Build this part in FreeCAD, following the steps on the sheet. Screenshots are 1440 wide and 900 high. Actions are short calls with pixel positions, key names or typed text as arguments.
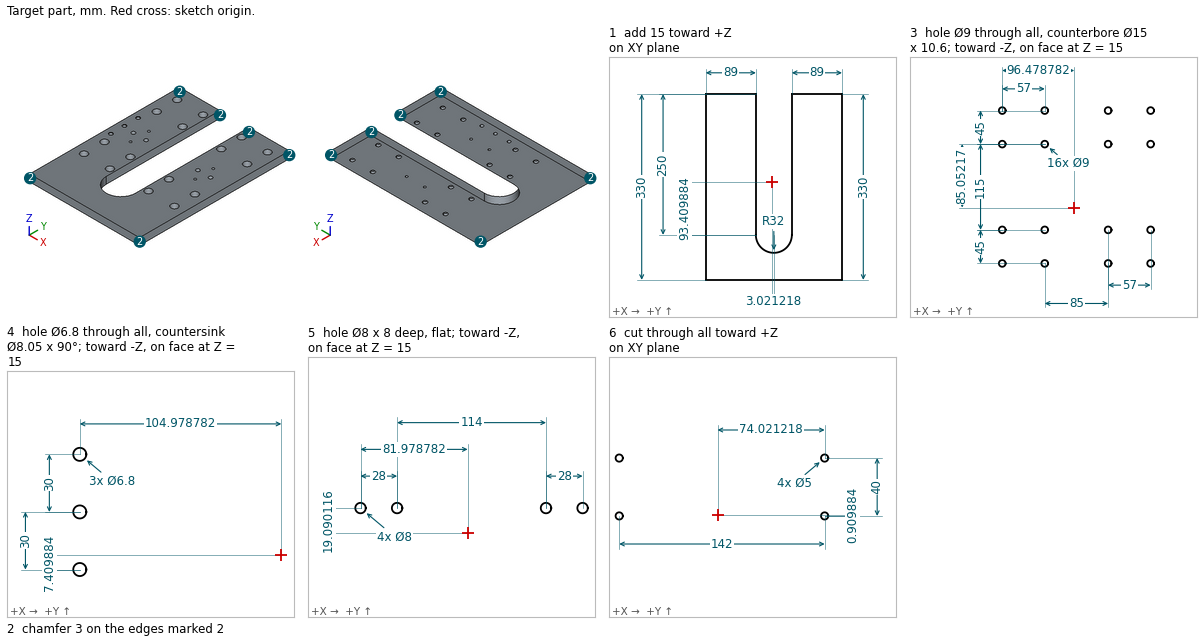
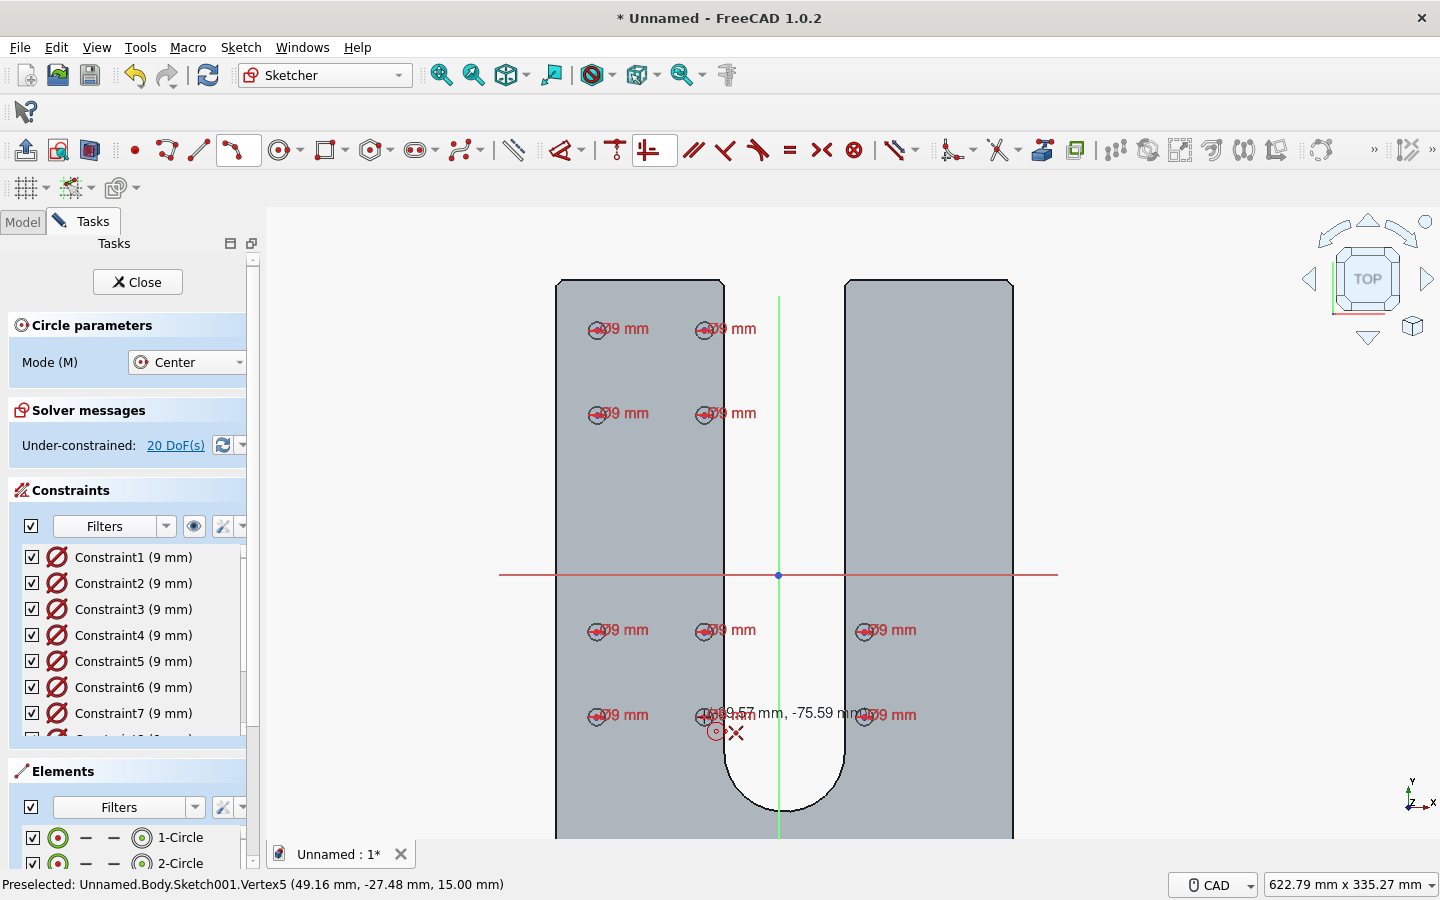
scroll(972, 632, up, 5)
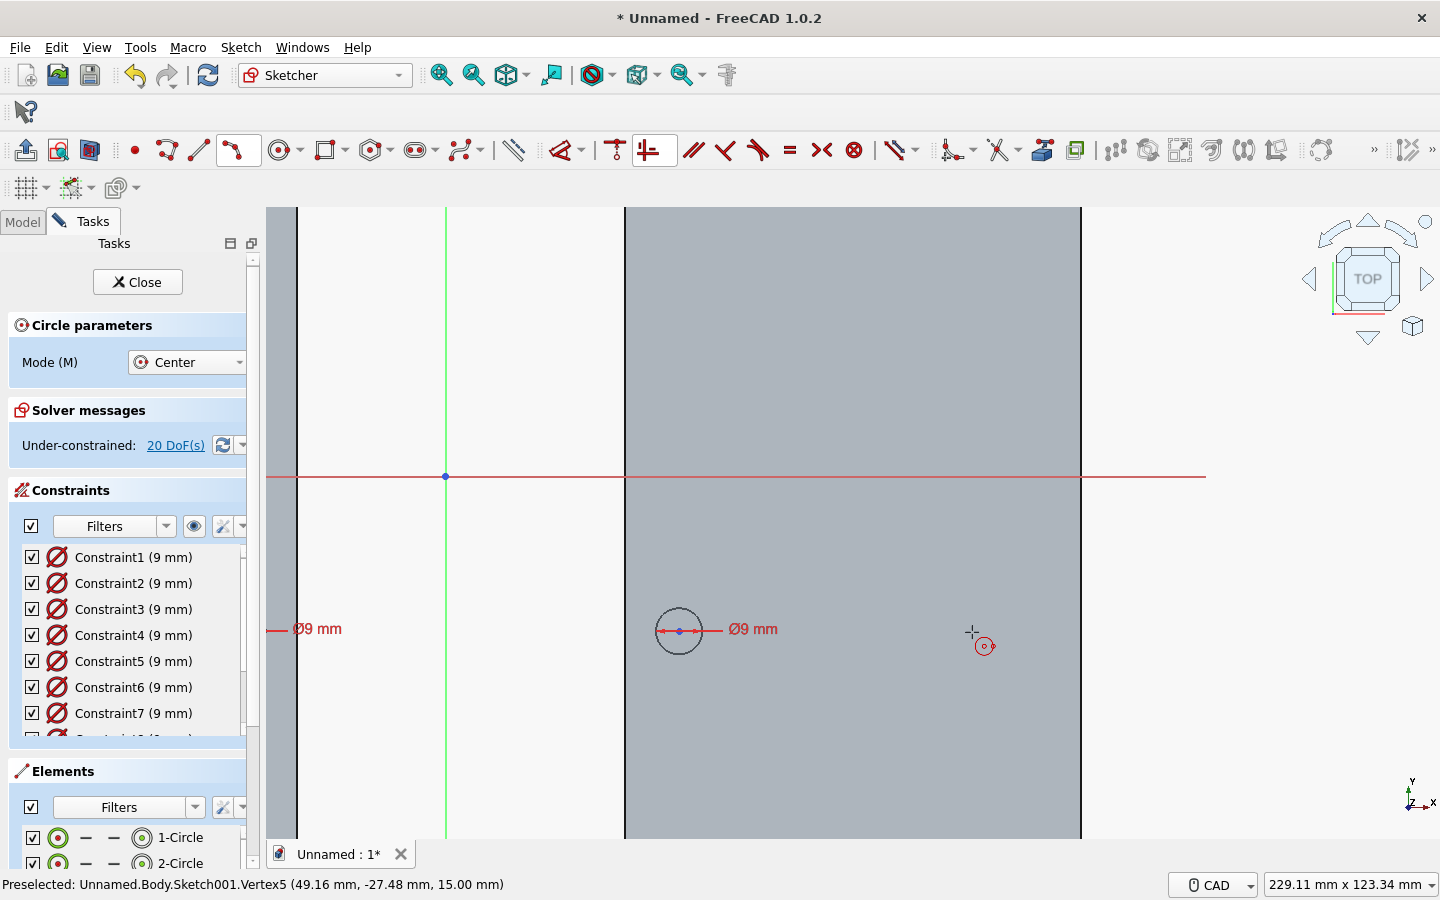
click(971, 630)
move(988, 614)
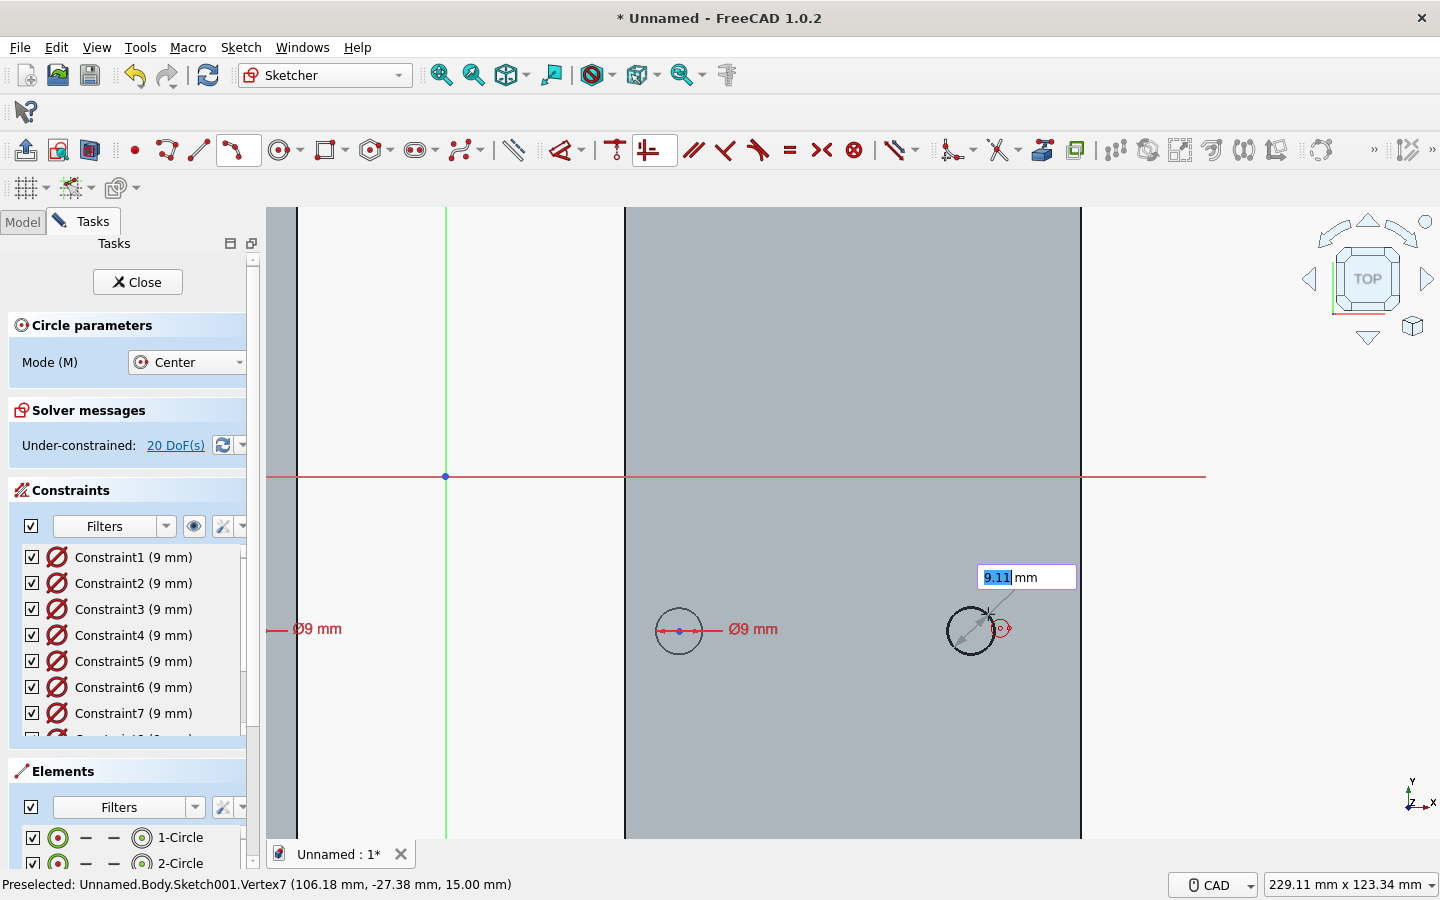
text(9)
key(Return)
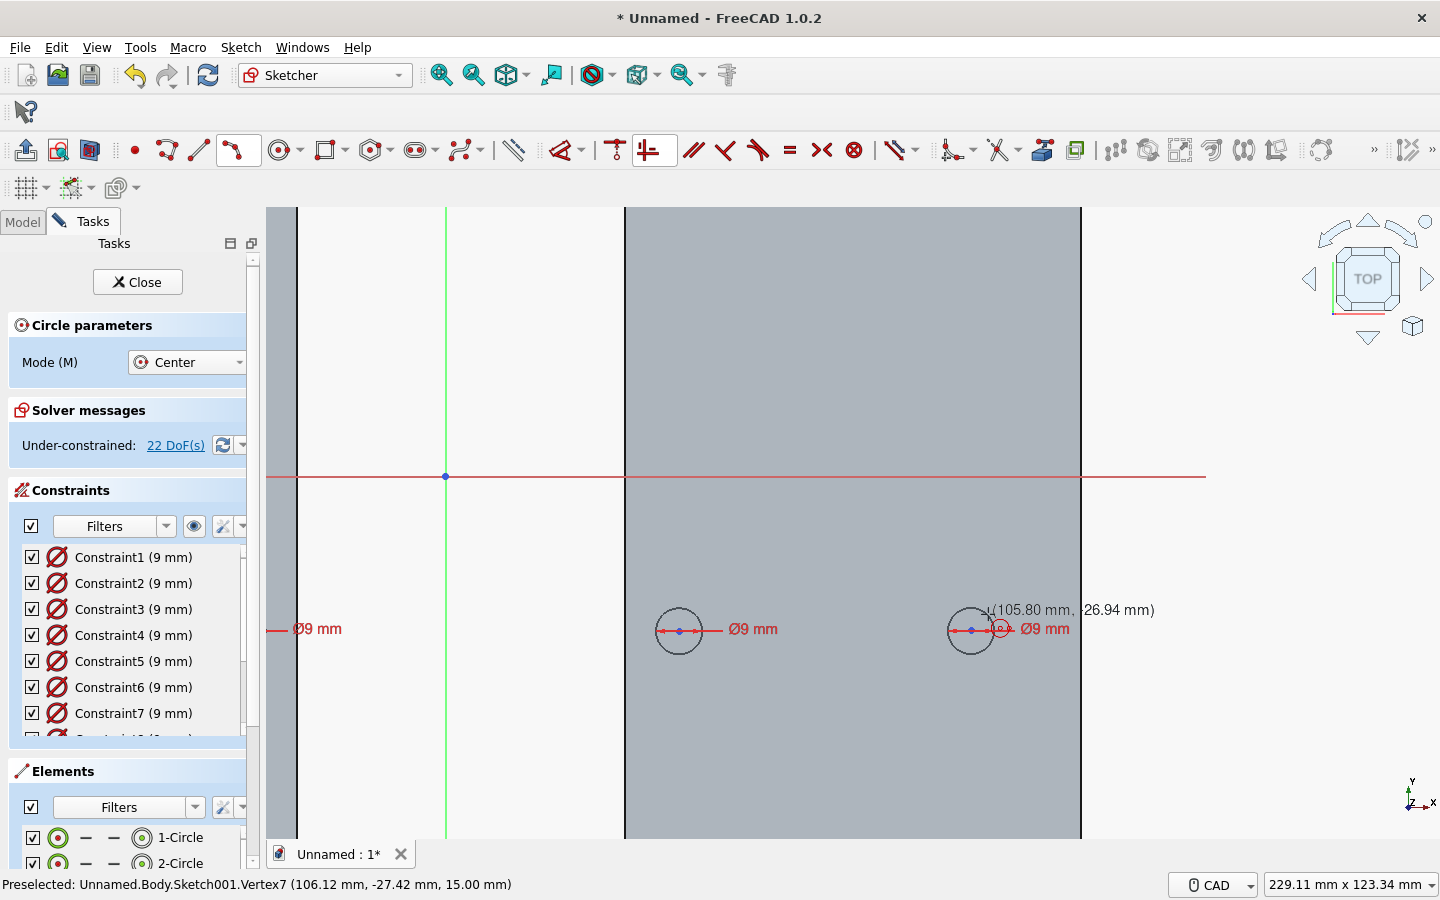
scroll(973, 632, down, 5)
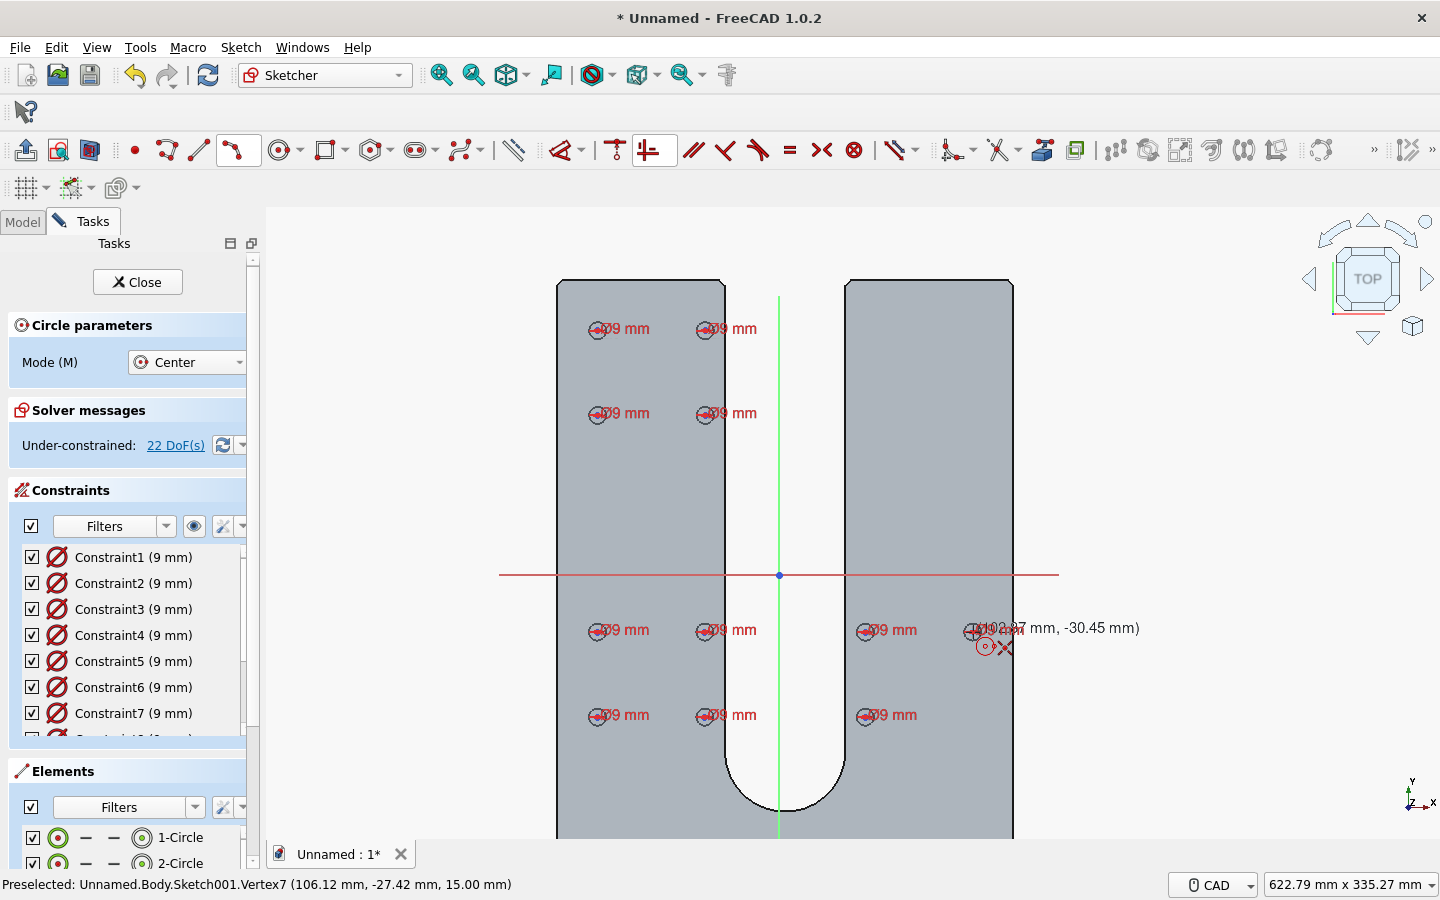
scroll(973, 717, up, 5)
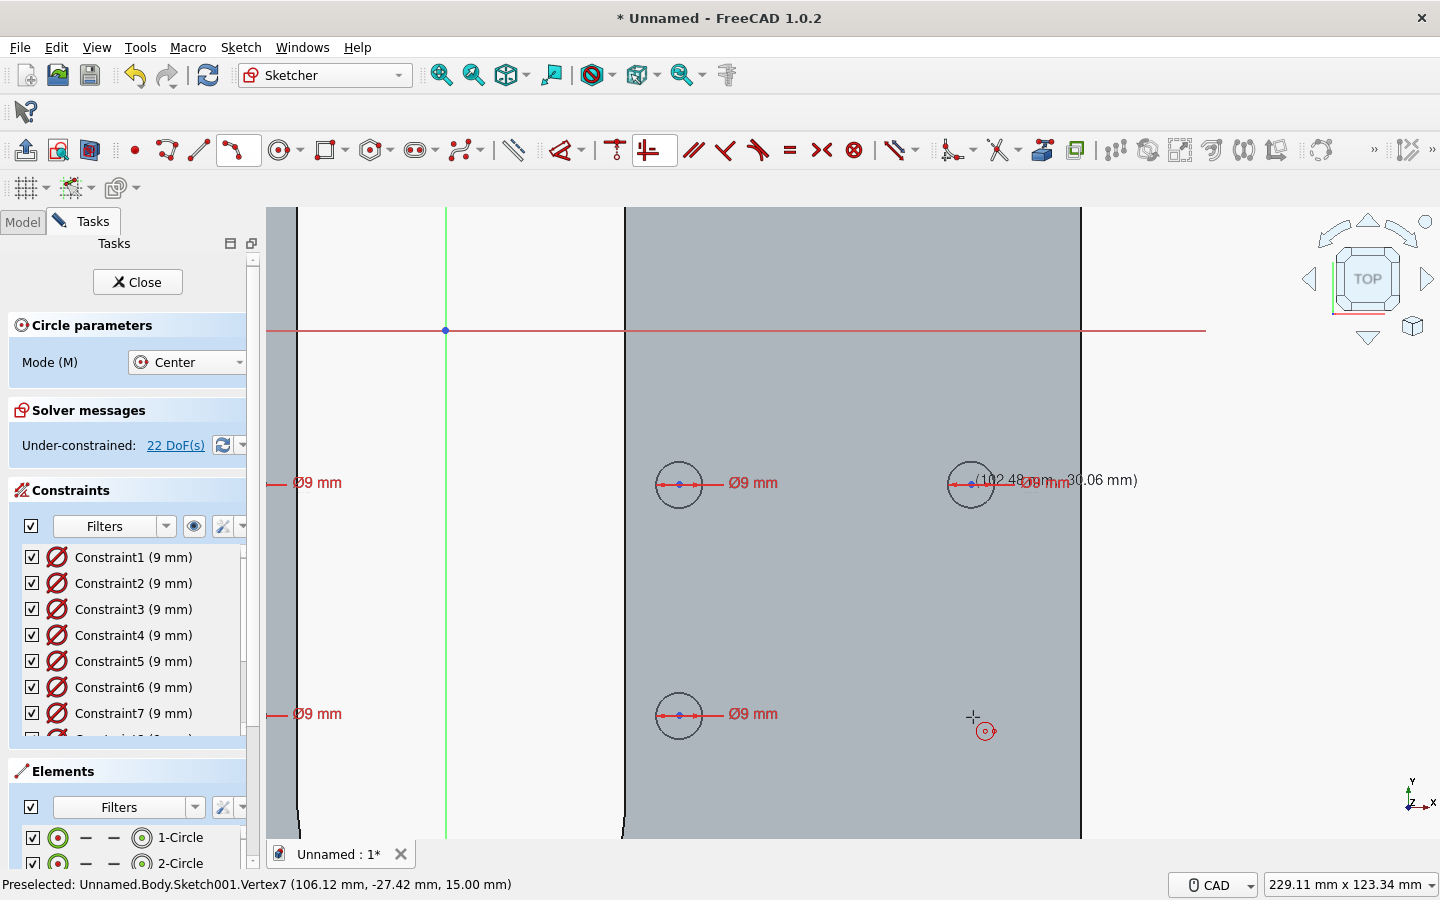
click(971, 715)
move(988, 698)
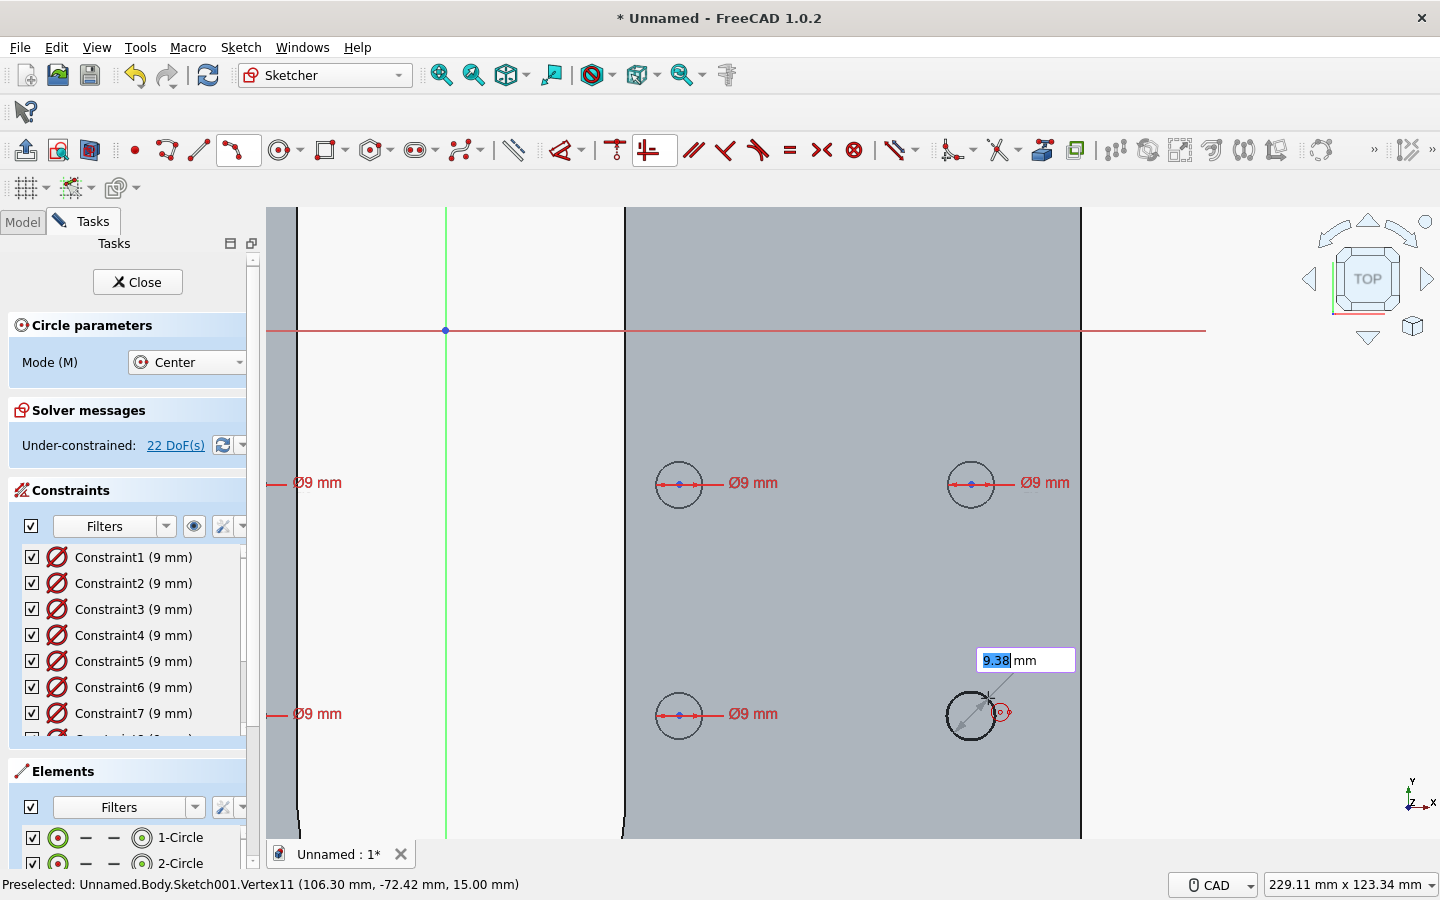
text(9)
key(Return)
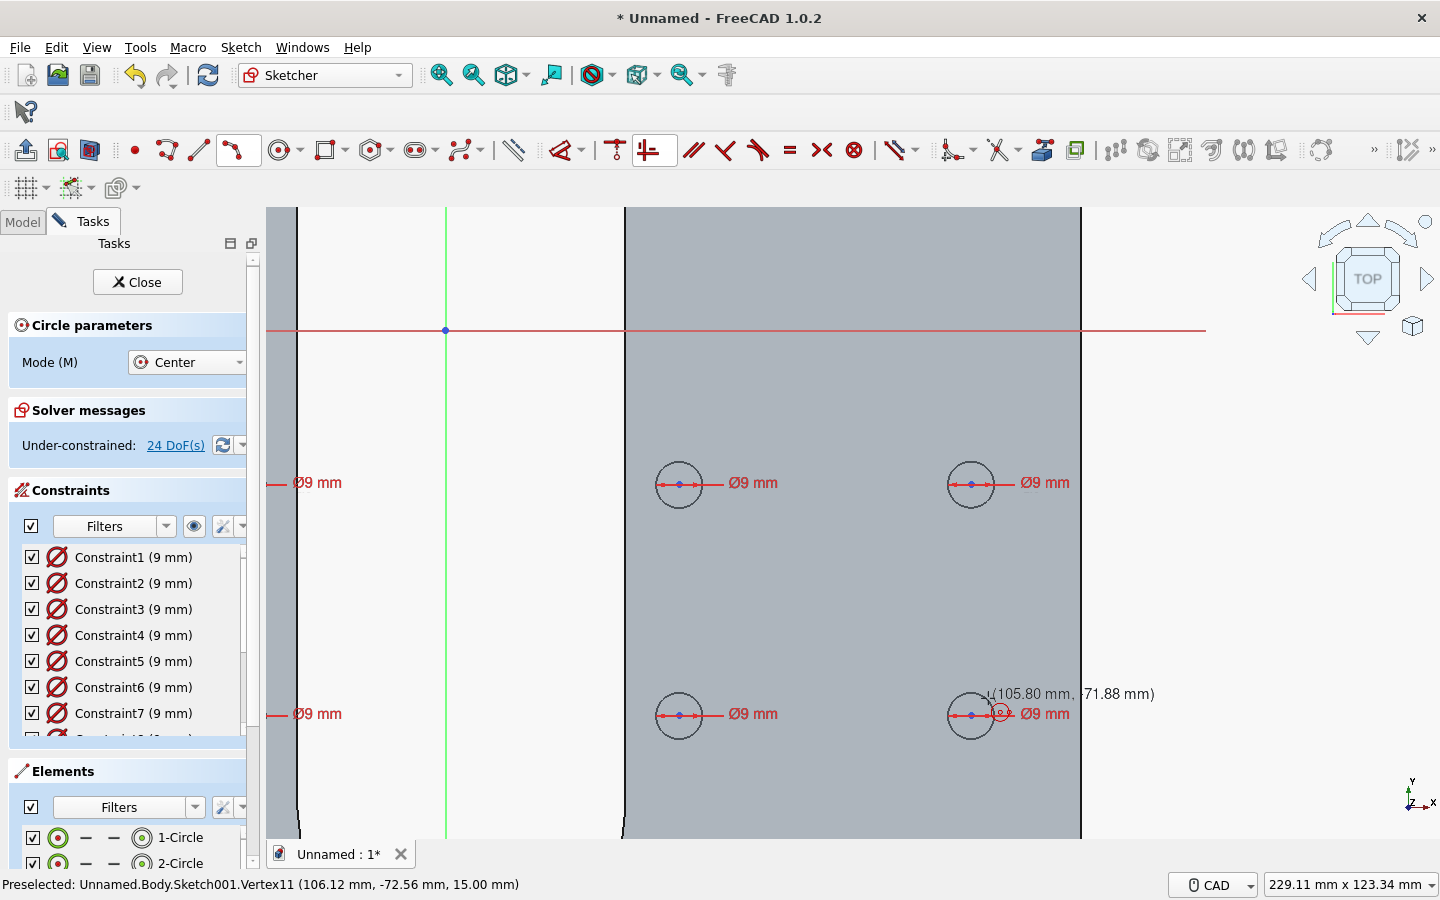
scroll(973, 717, down, 5)